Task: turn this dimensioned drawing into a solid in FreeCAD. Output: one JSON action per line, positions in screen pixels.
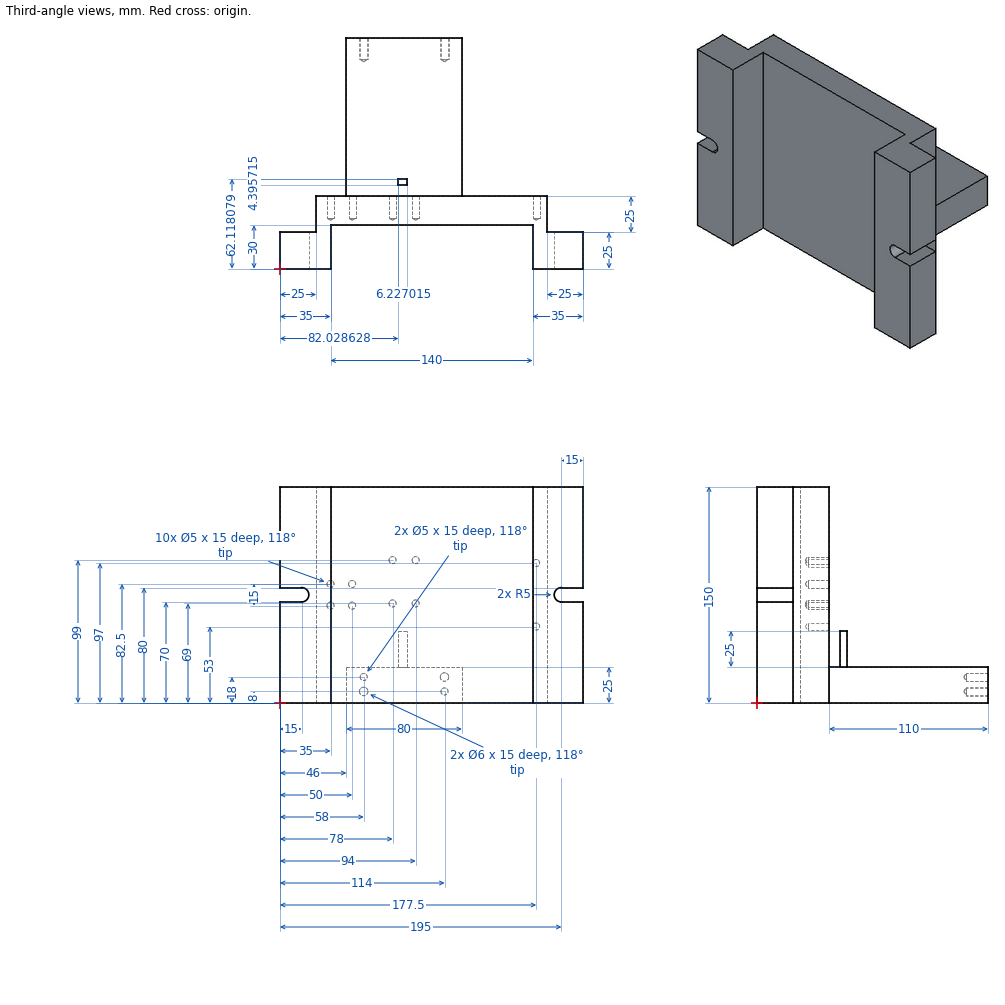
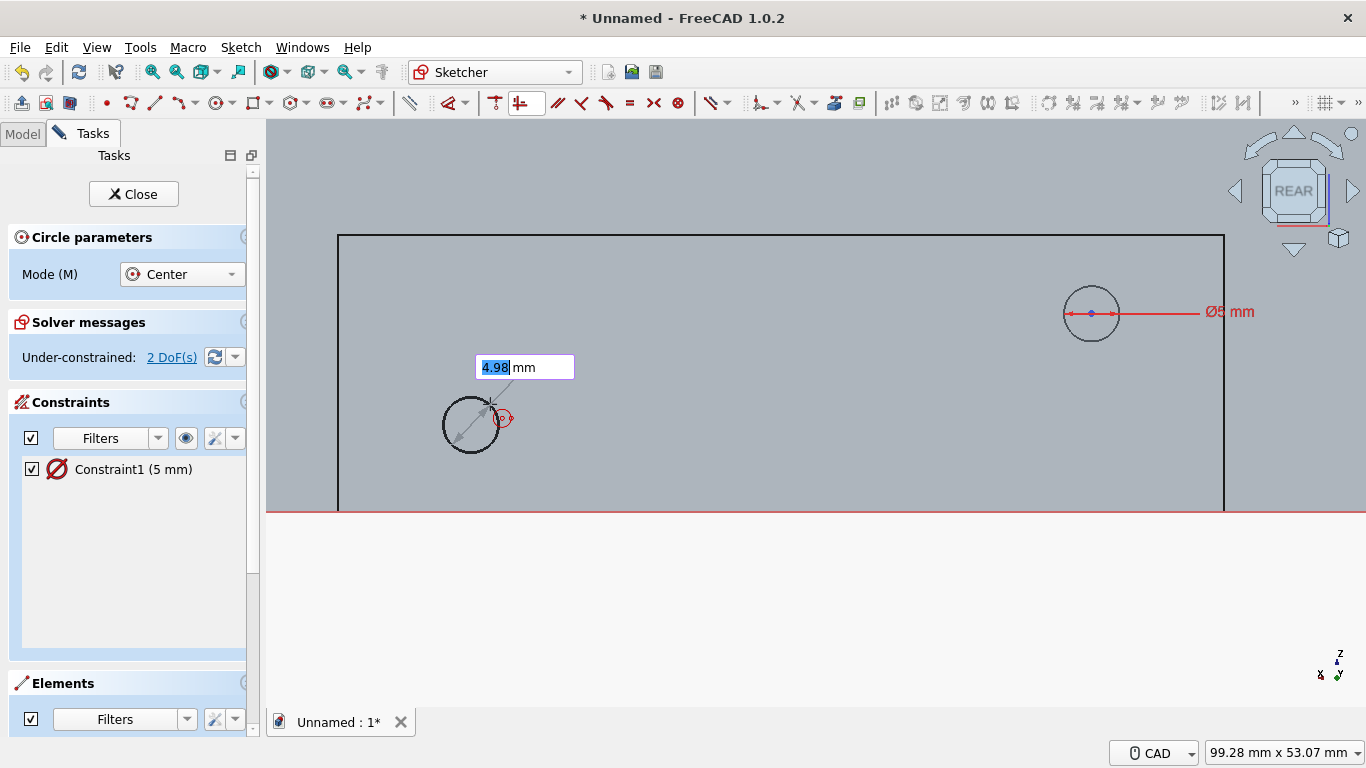
{"action": "type", "text": "5"}
{"action": "key", "text": "Return"}
{"action": "key", "text": "Escape"}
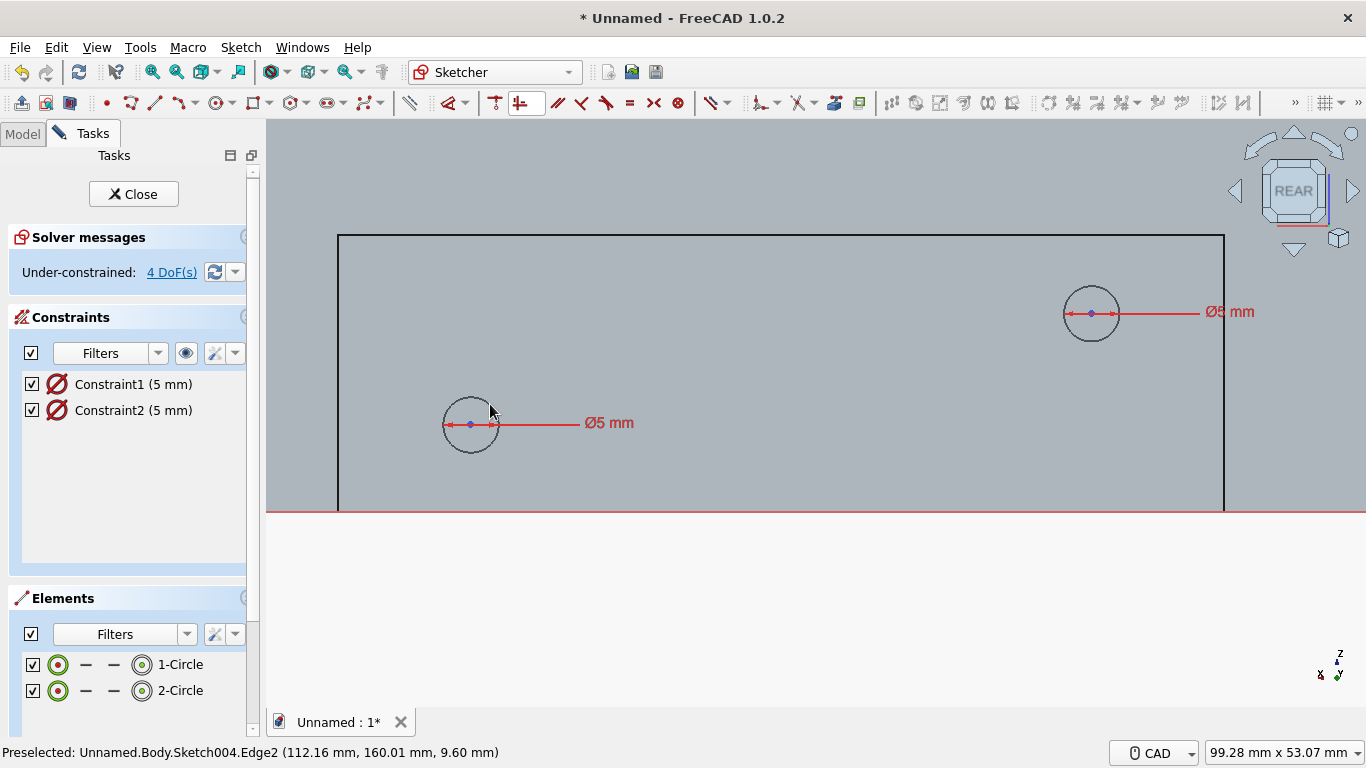
{"action": "key", "text": "d"}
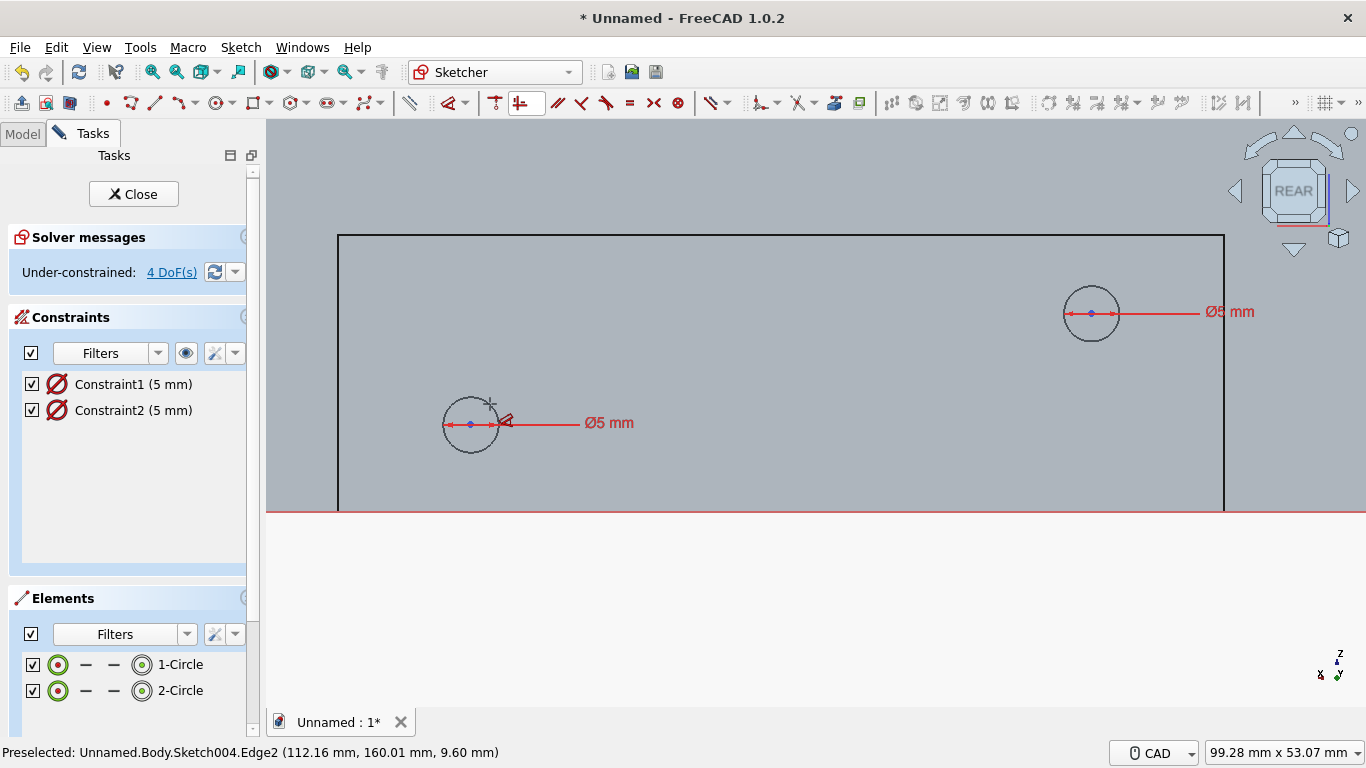
{"action": "left_click", "coordinate": [471, 425]}
{"action": "left_click", "coordinate": [437, 469]}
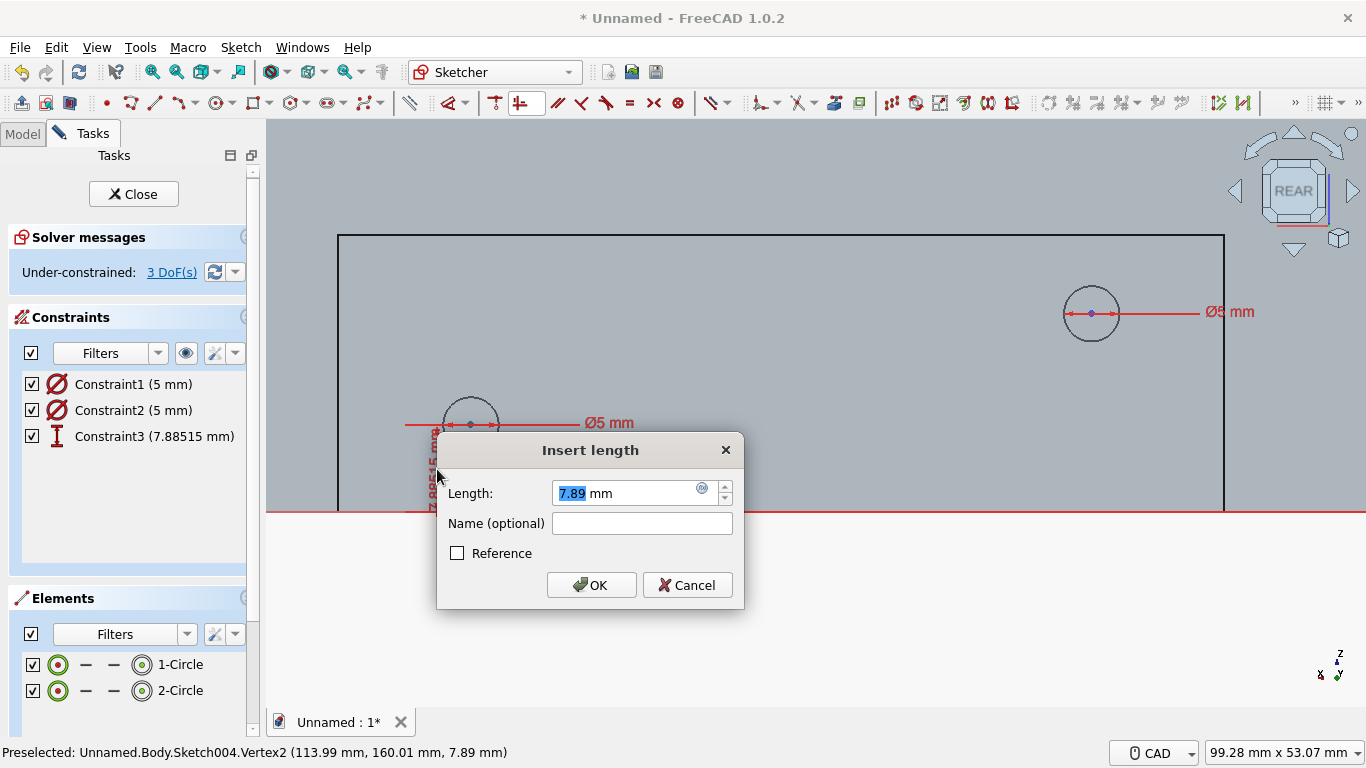
{"action": "type", "text": "8"}
{"action": "key", "text": "Return"}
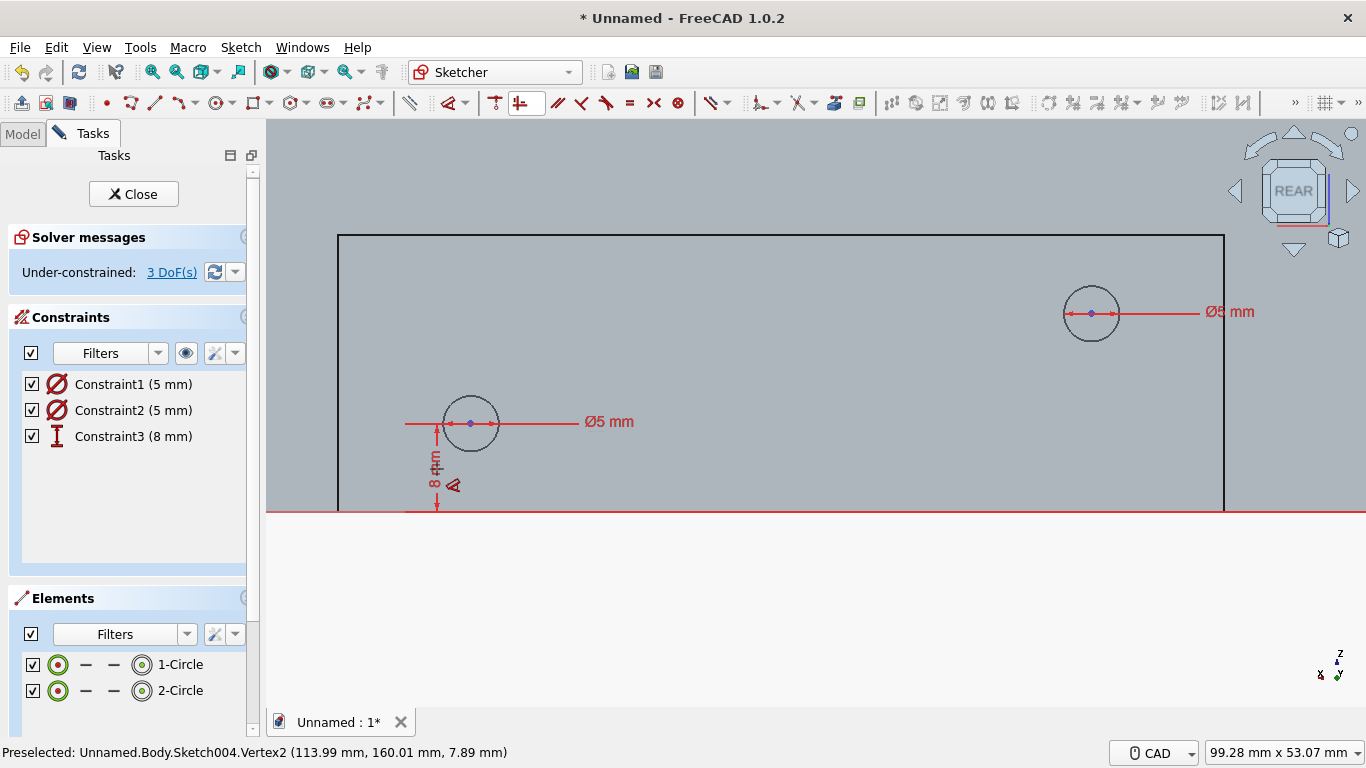
{"action": "left_click", "coordinate": [1092, 314]}
{"action": "left_click", "coordinate": [1146, 546]}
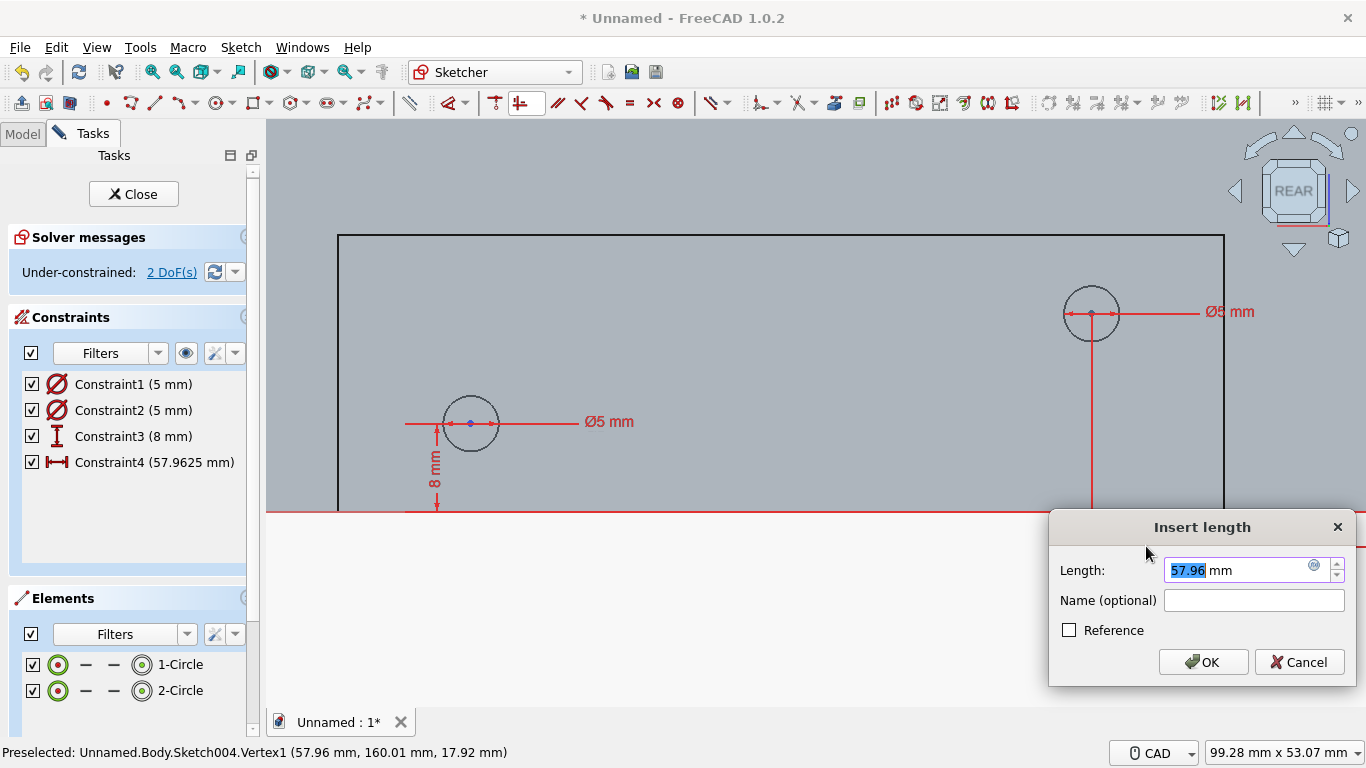
{"action": "type", "text": "58"}
{"action": "key", "text": "Return"}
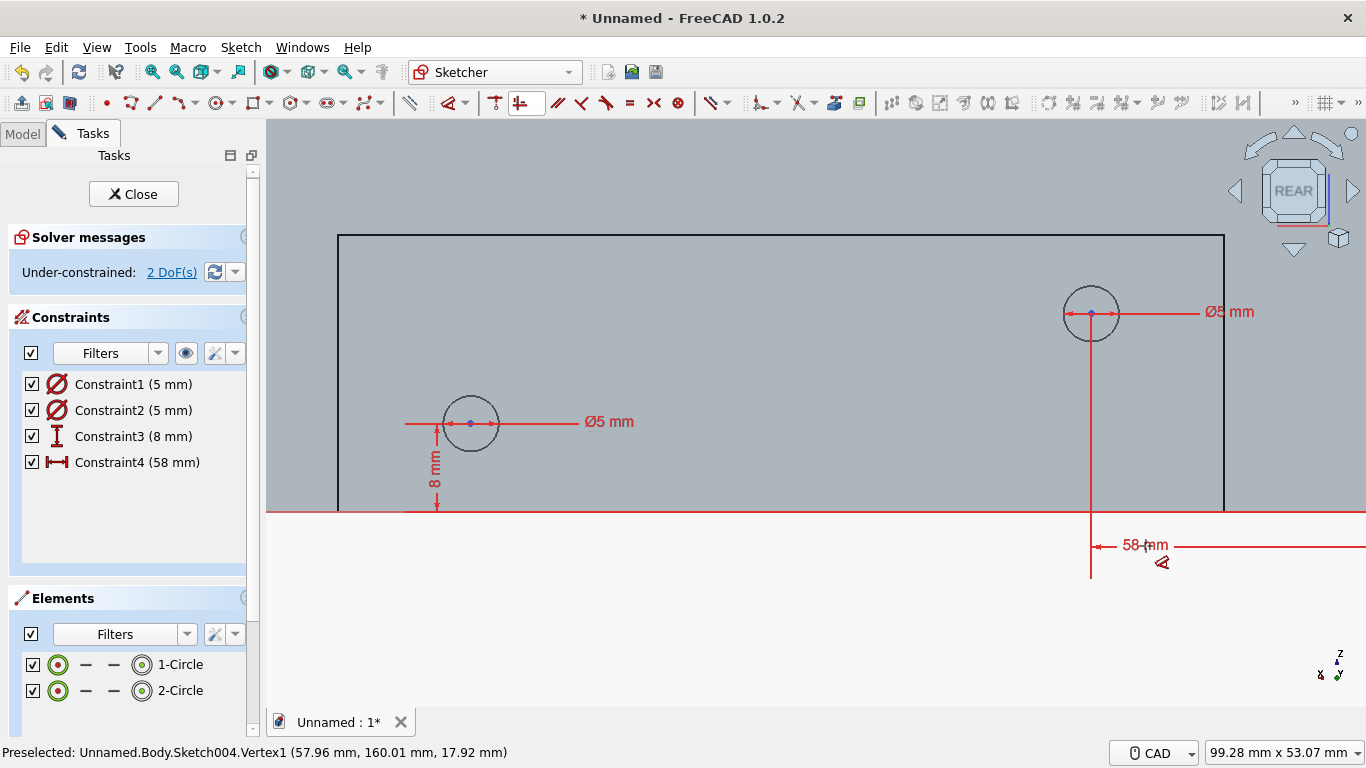
{"action": "left_click", "coordinate": [1091, 314]}
{"action": "left_click", "coordinate": [1057, 413]}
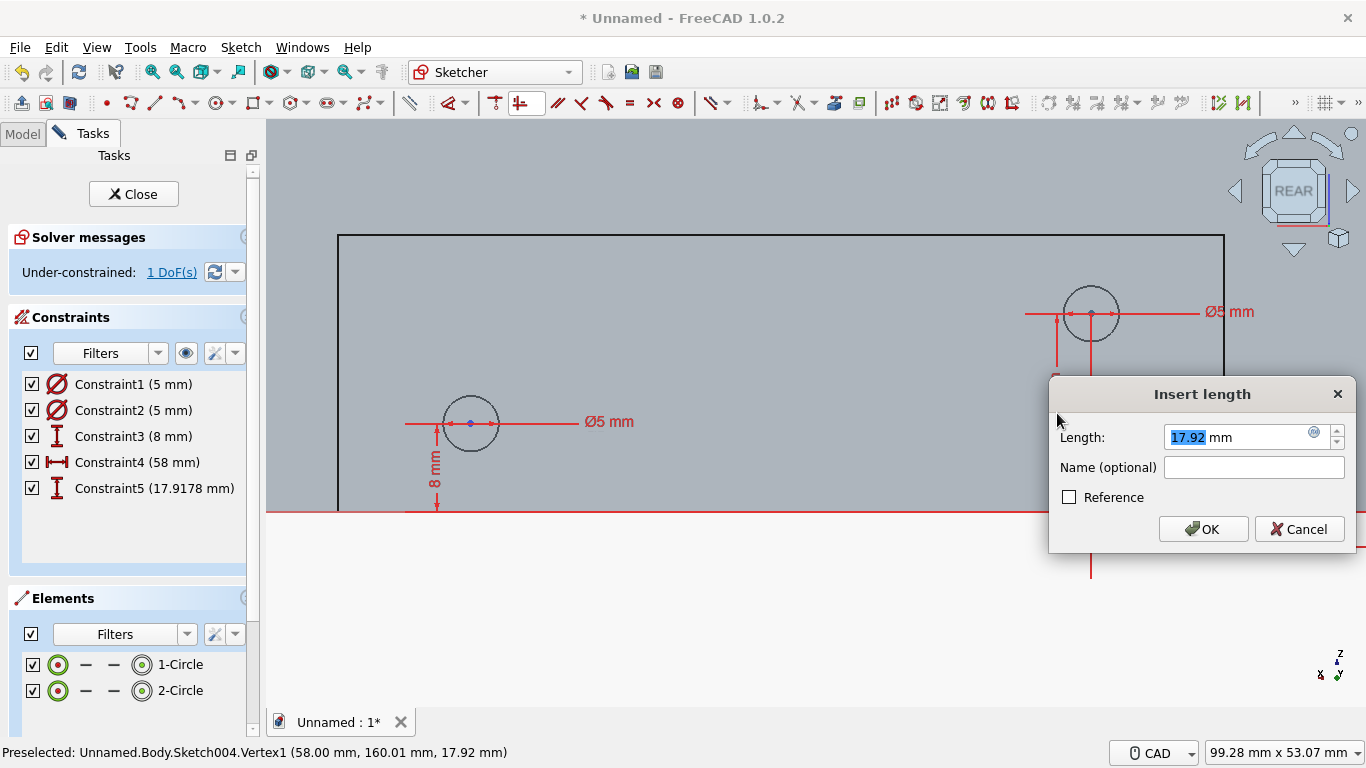
{"action": "type", "text": "18"}
{"action": "key", "text": "Return"}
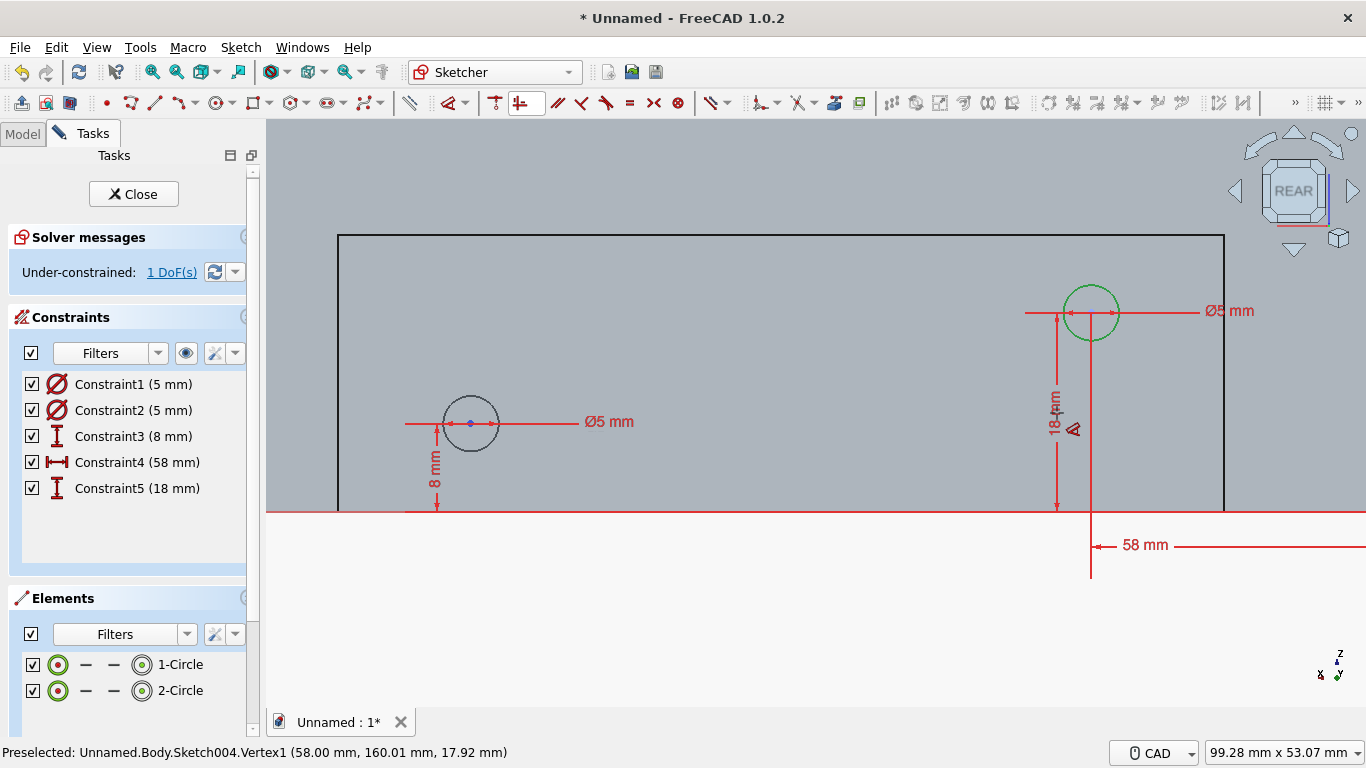
{"action": "left_click", "coordinate": [471, 424]}
{"action": "left_click", "coordinate": [836, 546]}